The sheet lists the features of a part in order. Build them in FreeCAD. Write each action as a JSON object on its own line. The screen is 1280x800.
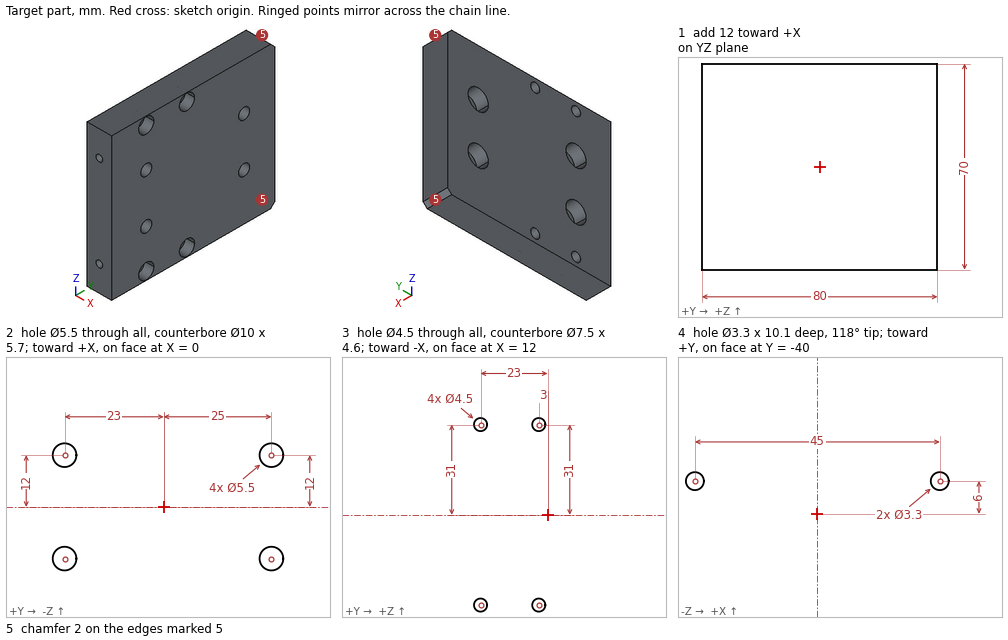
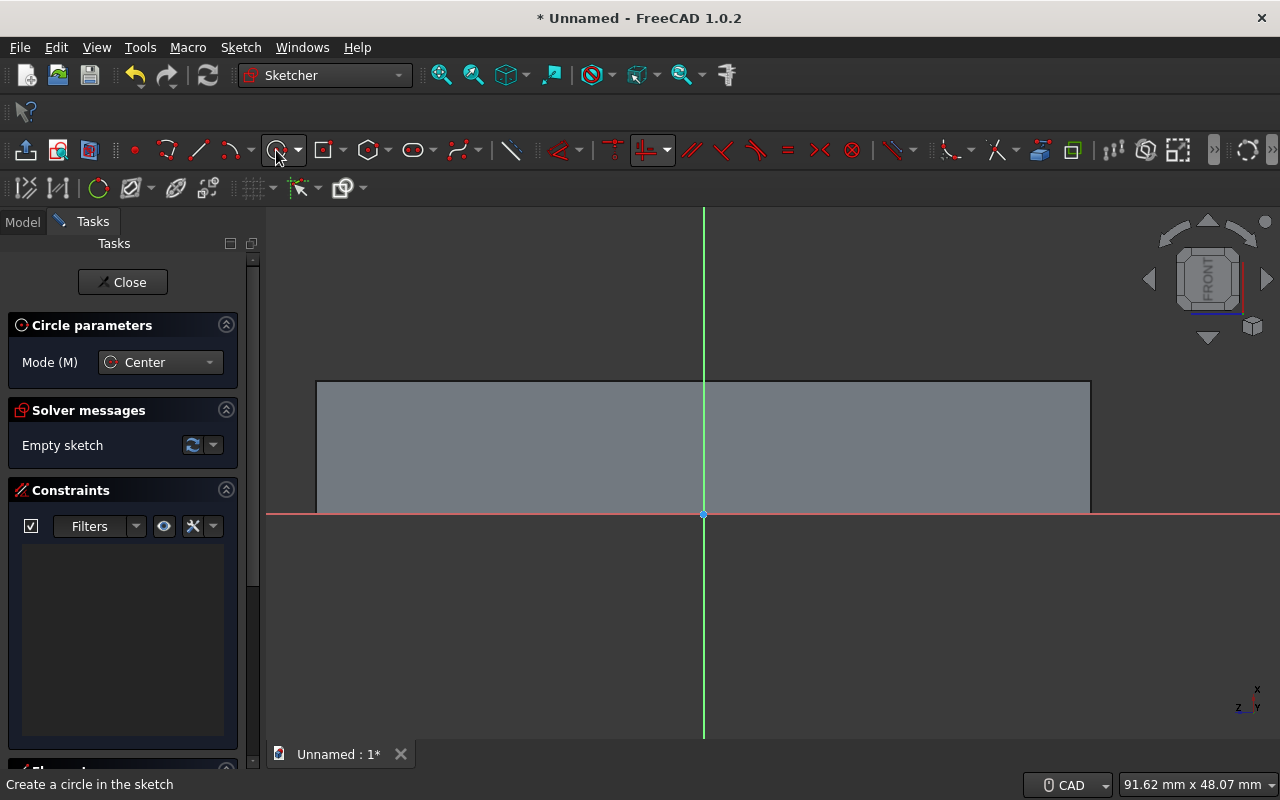
{"action": "scroll", "coordinate": [953, 448], "scroll_direction": "up", "scroll_amount": 2}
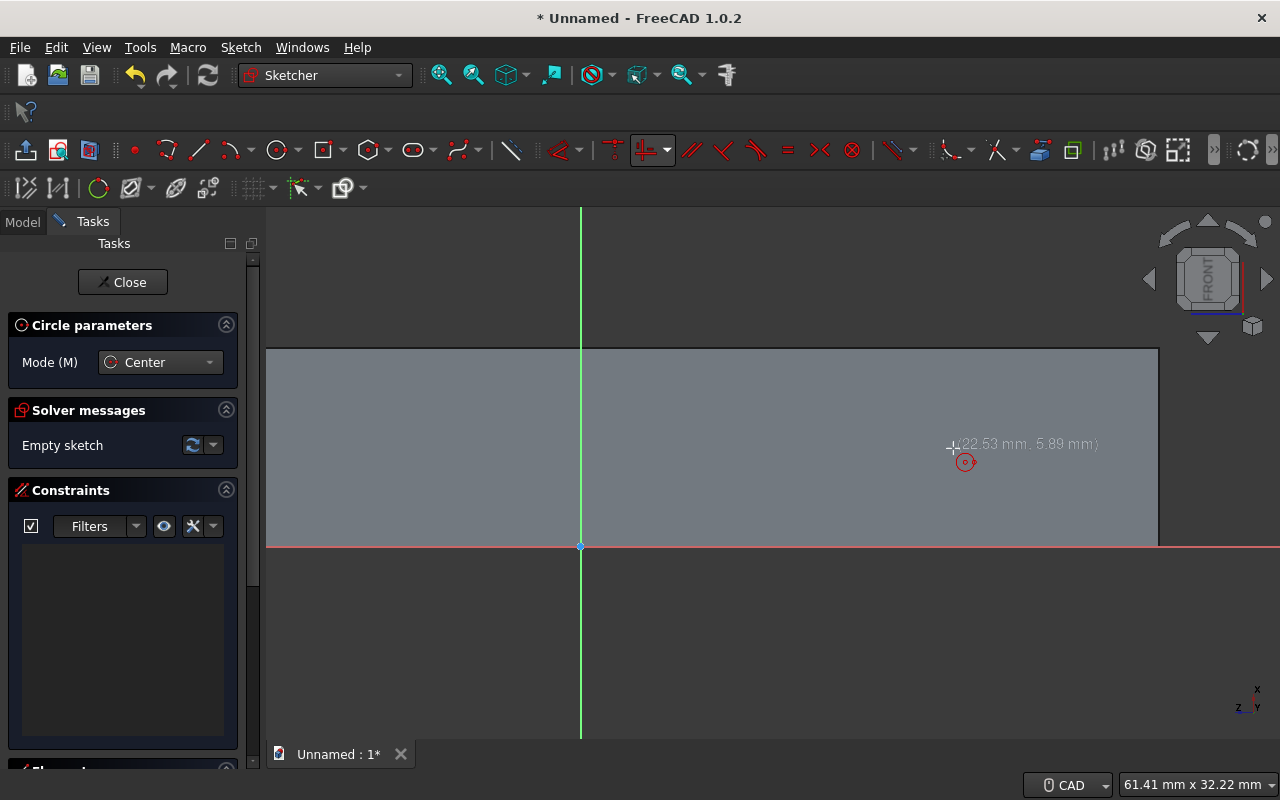
{"action": "left_click", "coordinate": [952, 448]}
{"action": "left_click", "coordinate": [972, 428]}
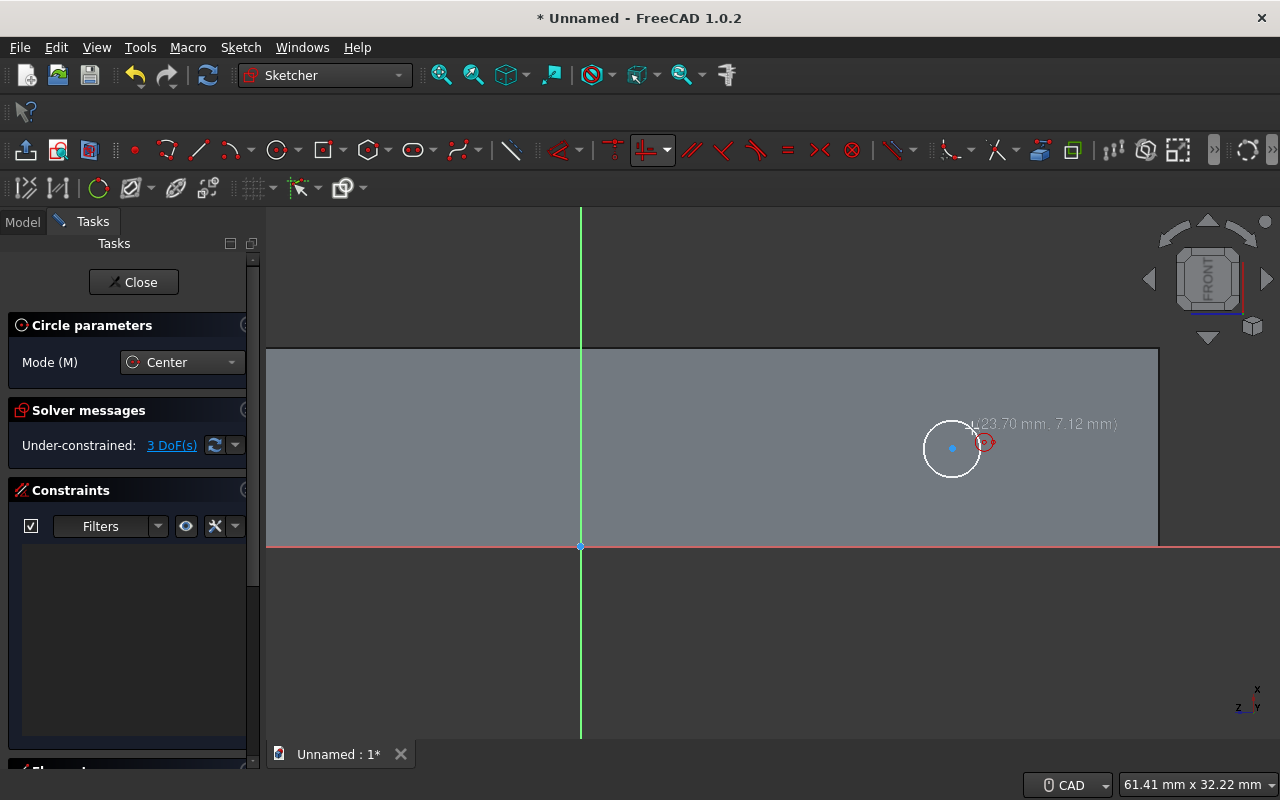
{"action": "scroll", "coordinate": [956, 452], "scroll_direction": "down", "scroll_amount": 2}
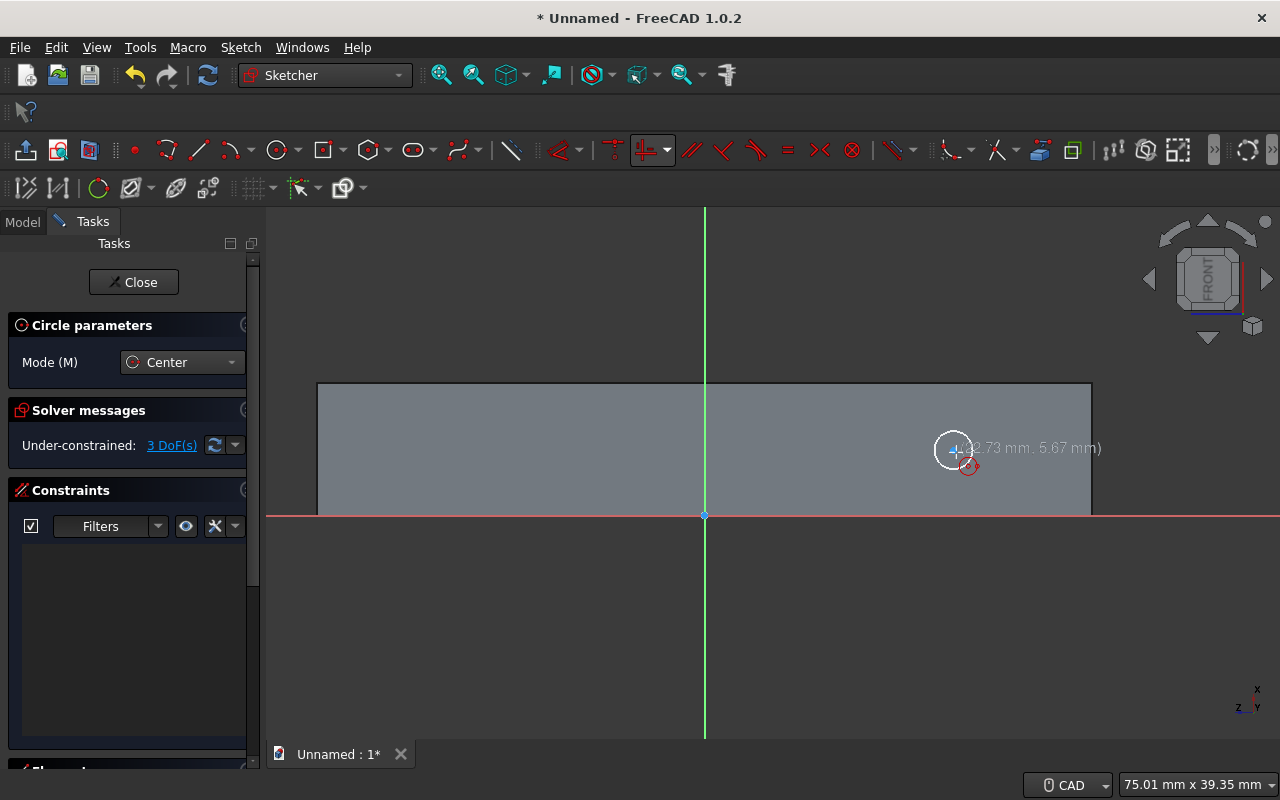
{"action": "scroll", "coordinate": [456, 449], "scroll_direction": "up", "scroll_amount": 2}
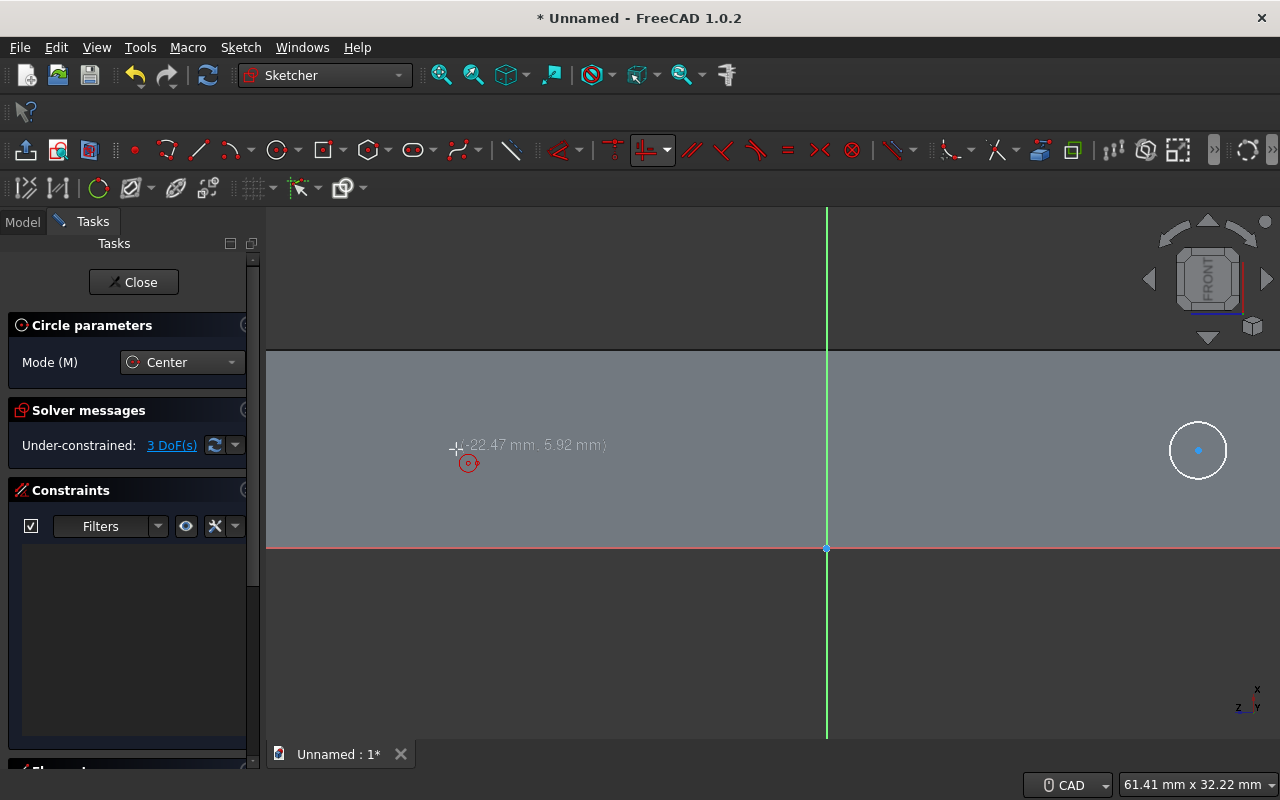
{"action": "left_click", "coordinate": [455, 449]}
{"action": "left_click", "coordinate": [475, 430]}
{"action": "key", "text": "Escape"}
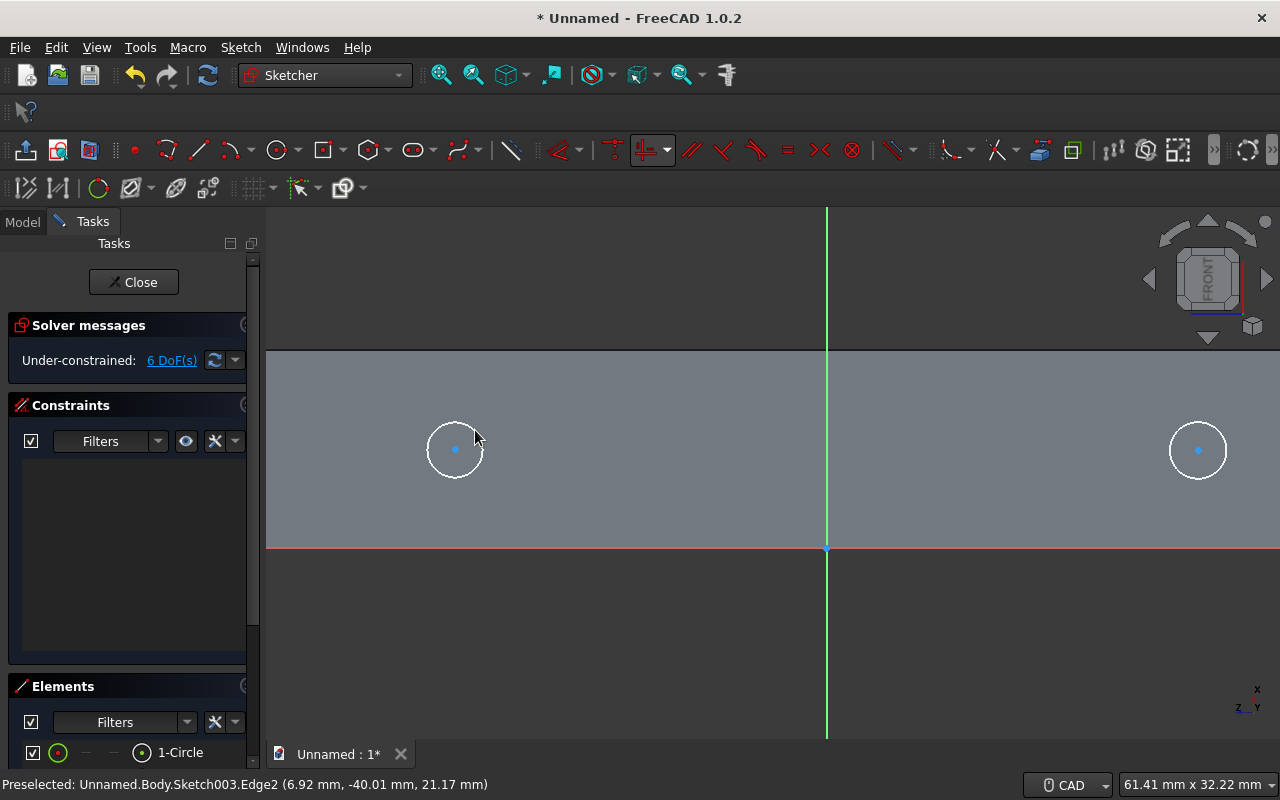
{"action": "scroll", "coordinate": [456, 449], "scroll_direction": "down", "scroll_amount": 2}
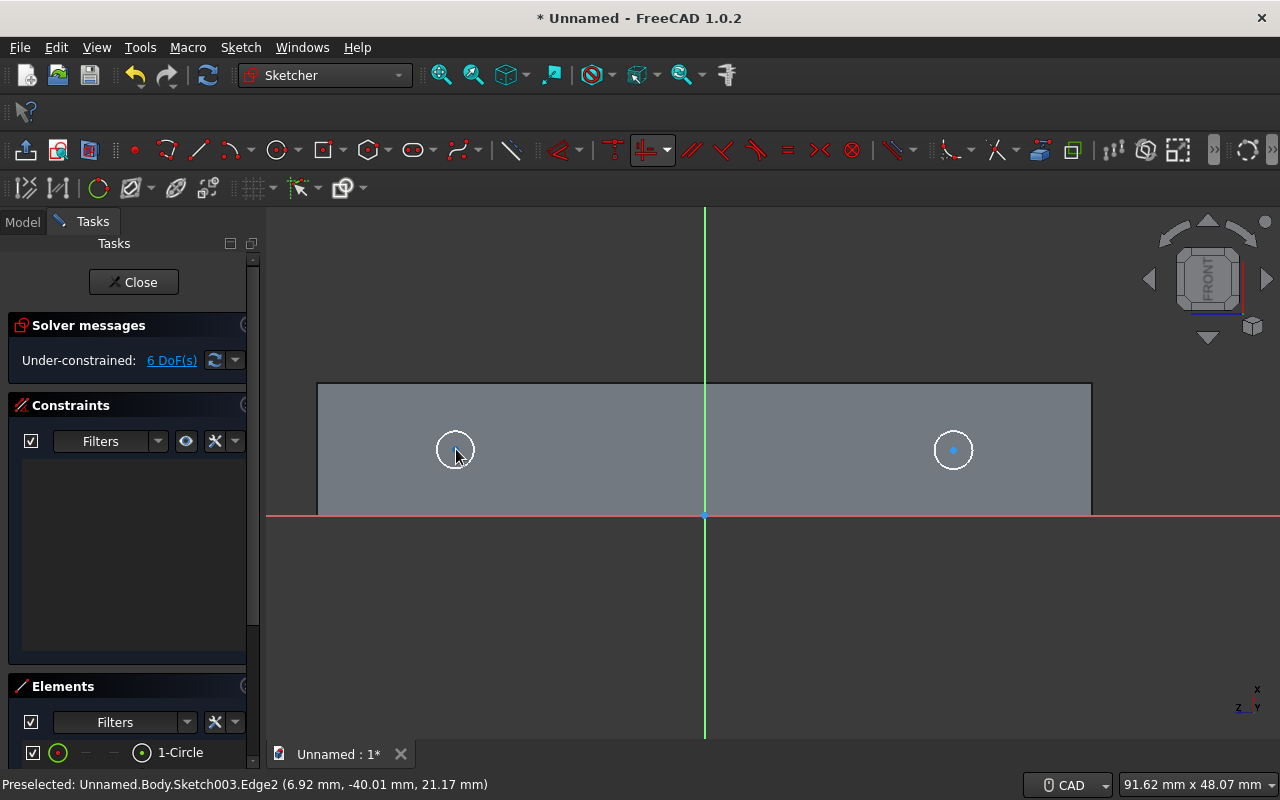
{"action": "left_click", "coordinate": [967, 437]}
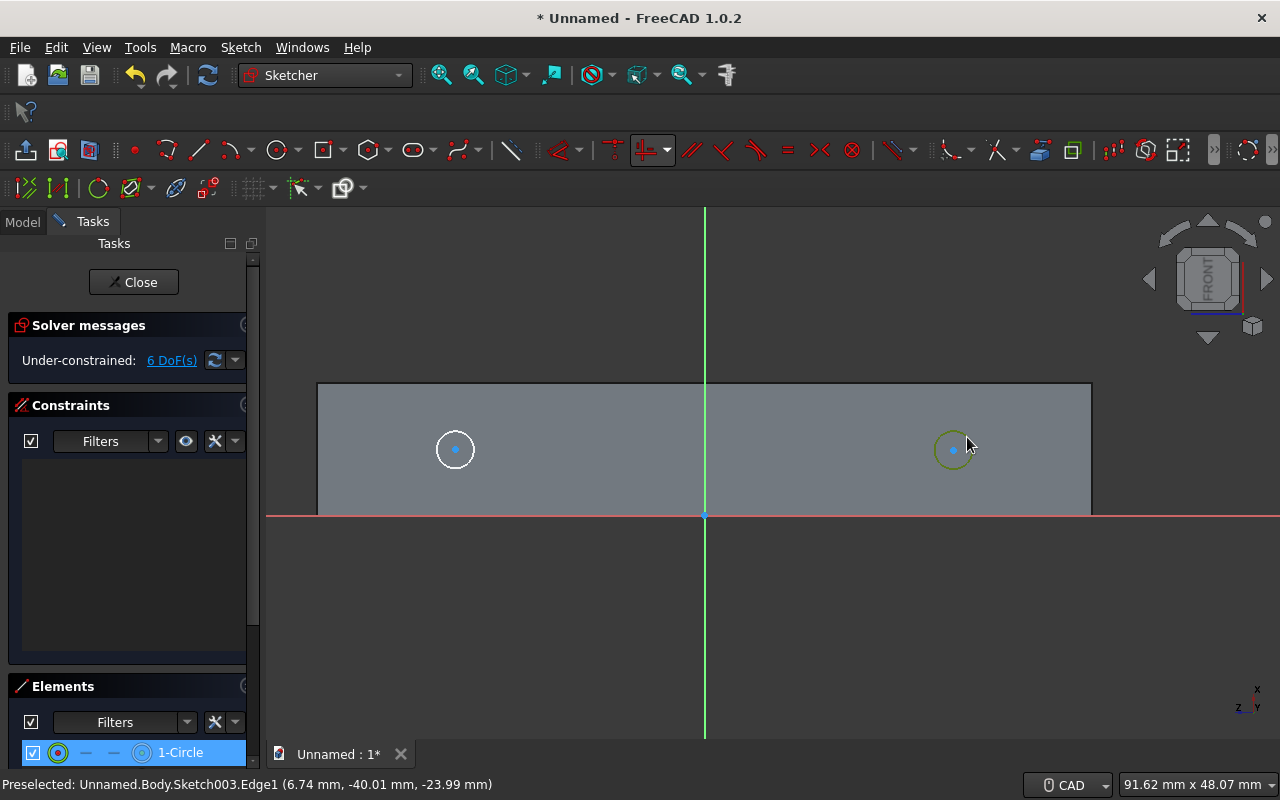
{"action": "left_click", "coordinate": [468, 437]}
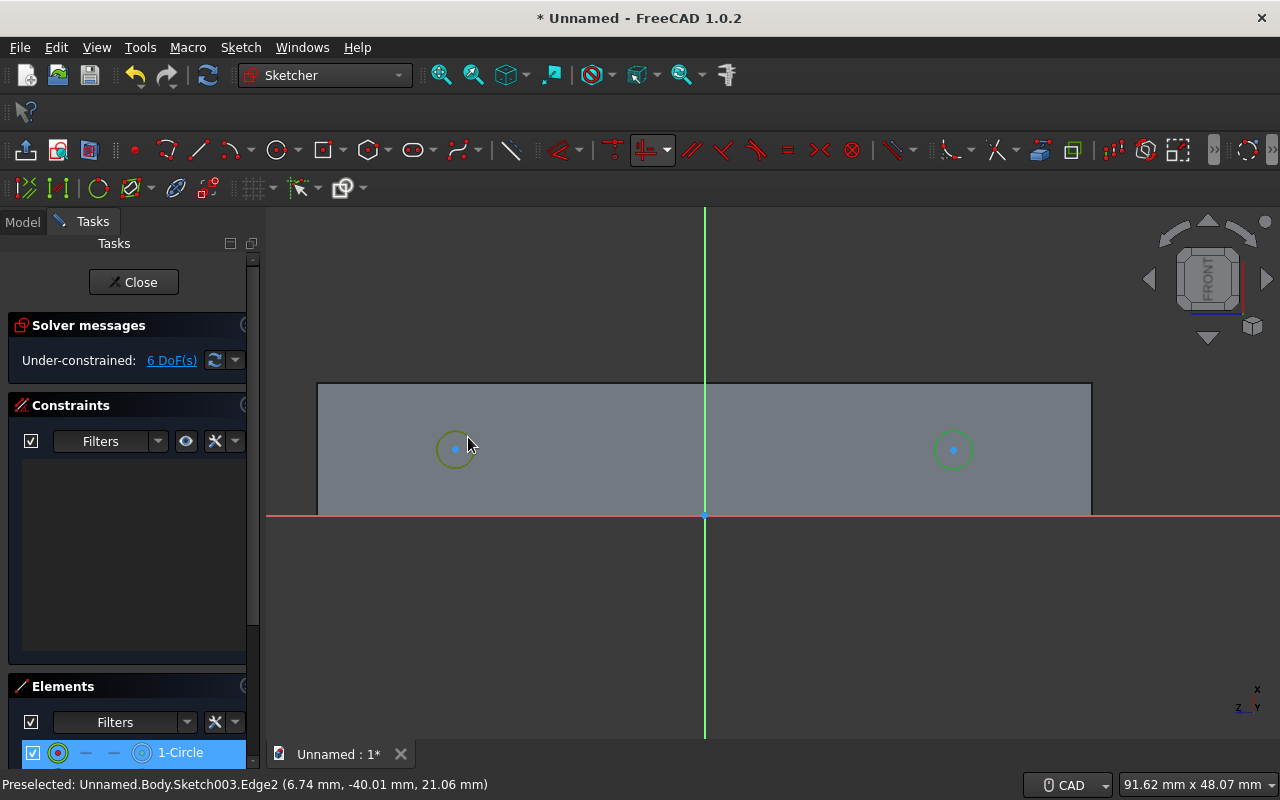
{"action": "left_click", "coordinate": [788, 150]}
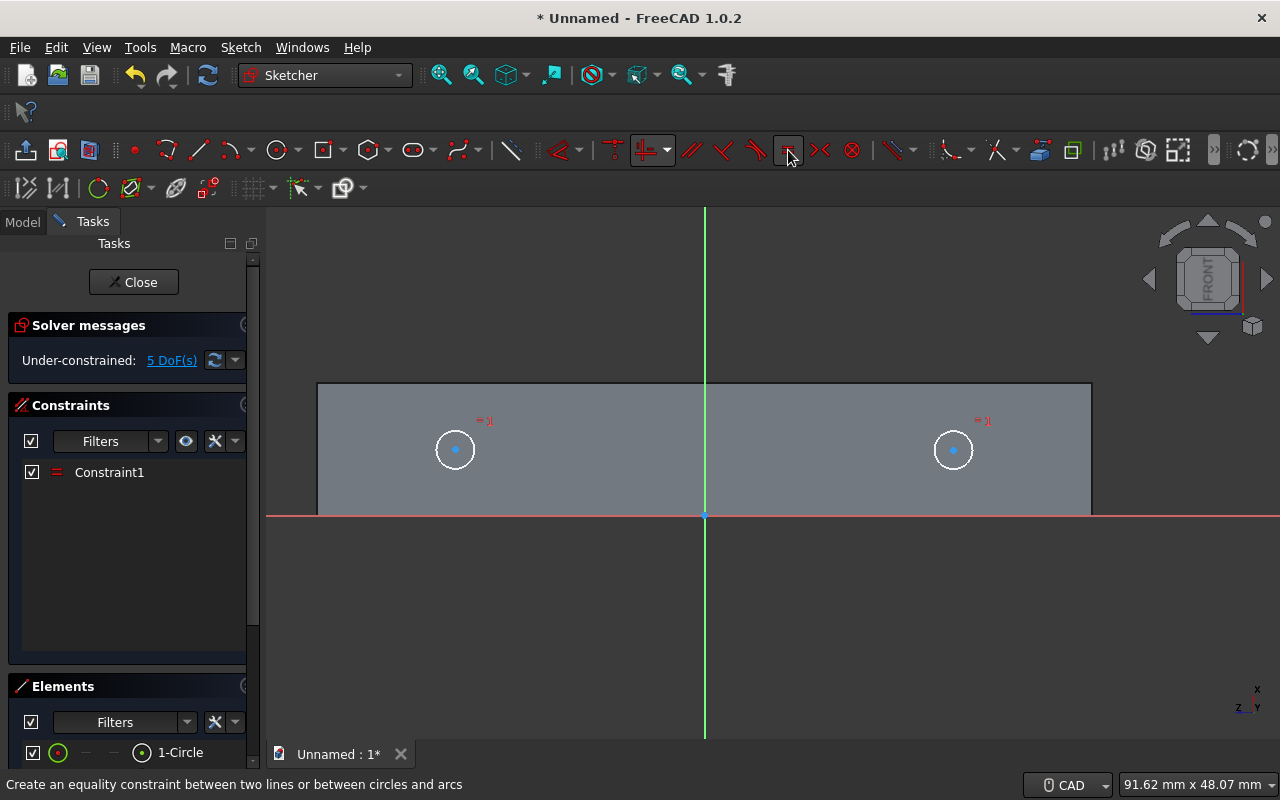
{"action": "left_click", "coordinate": [954, 450]}